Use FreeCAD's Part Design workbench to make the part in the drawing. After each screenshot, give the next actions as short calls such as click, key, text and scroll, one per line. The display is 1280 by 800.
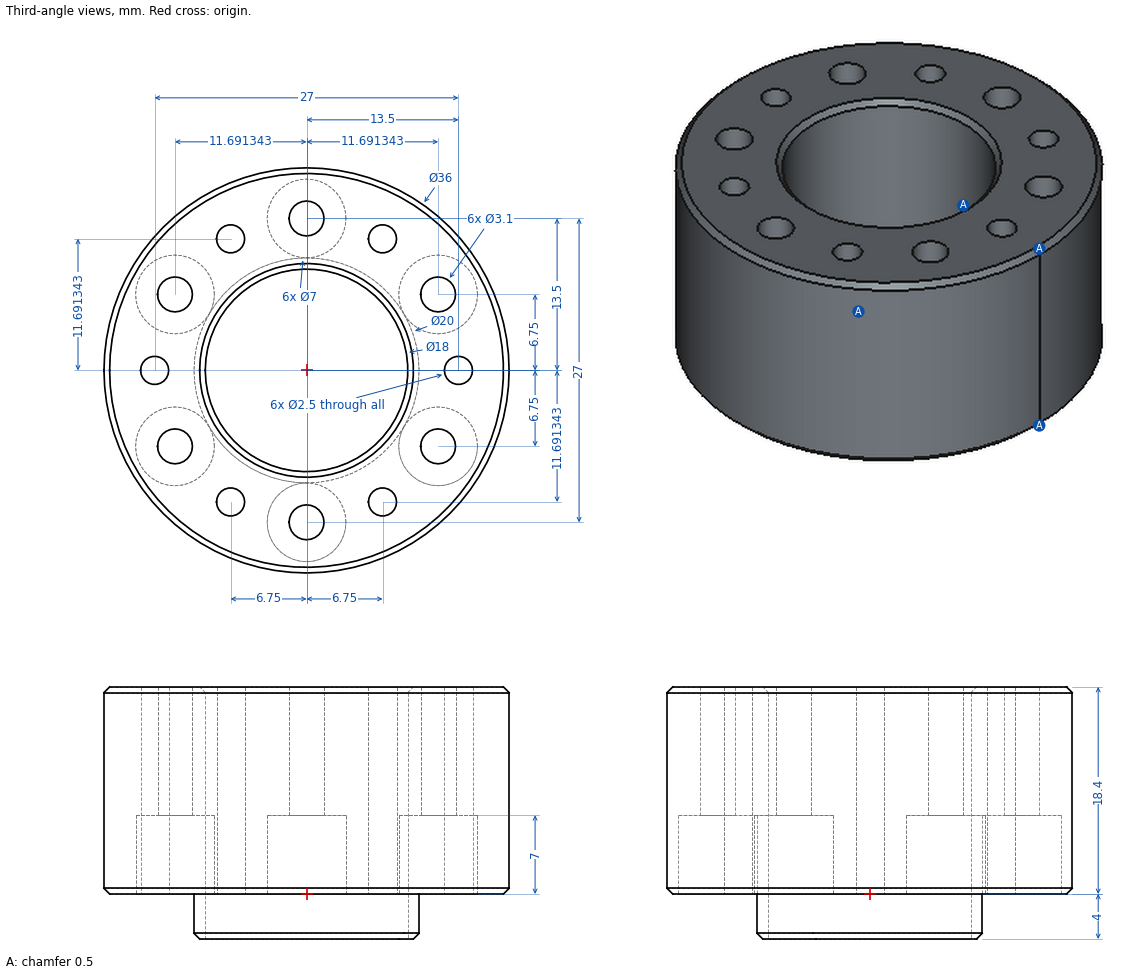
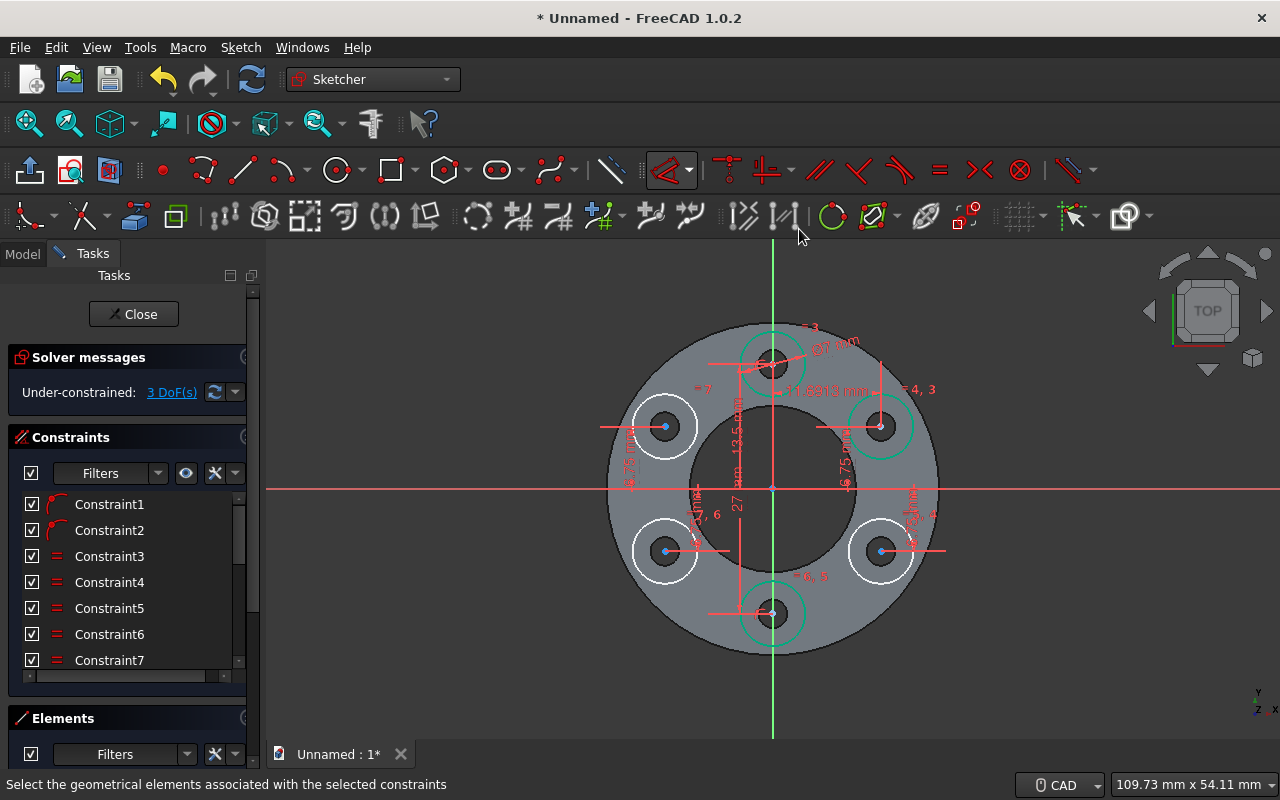
click(881, 551)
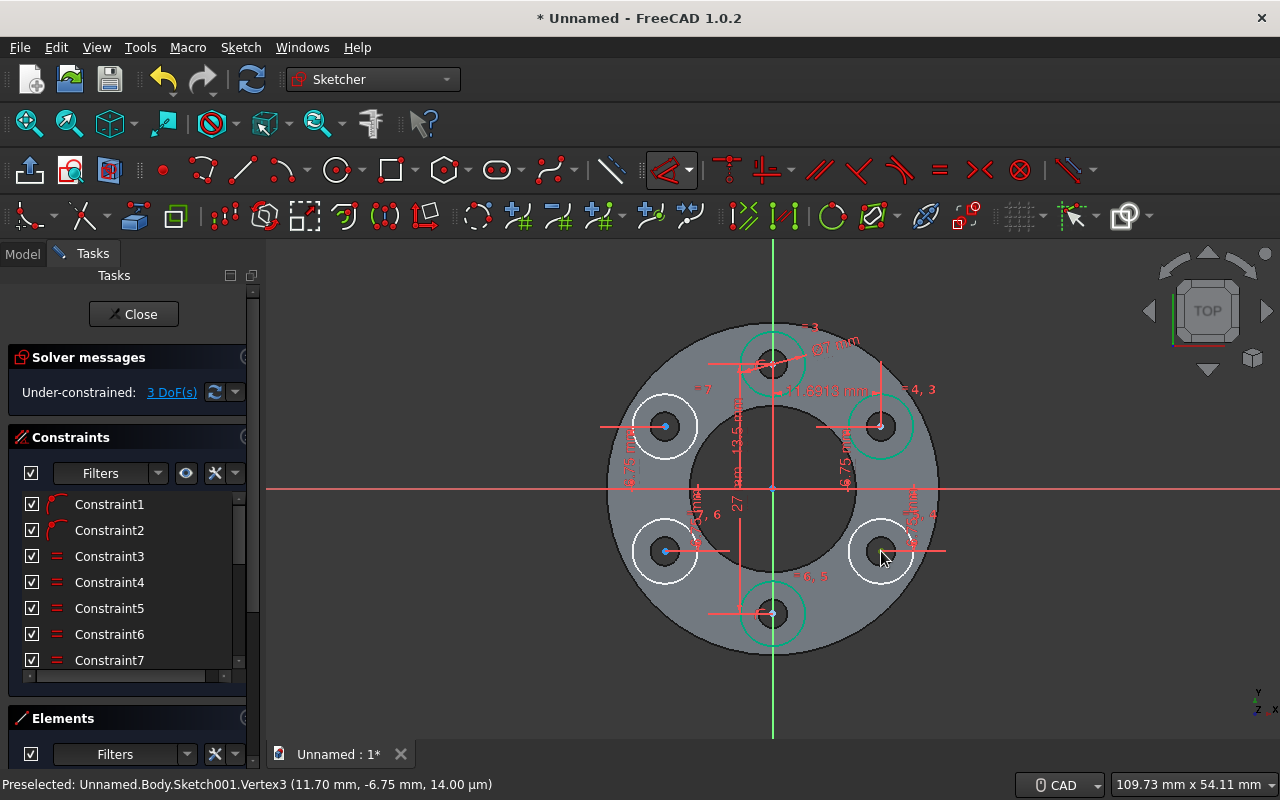
key(l)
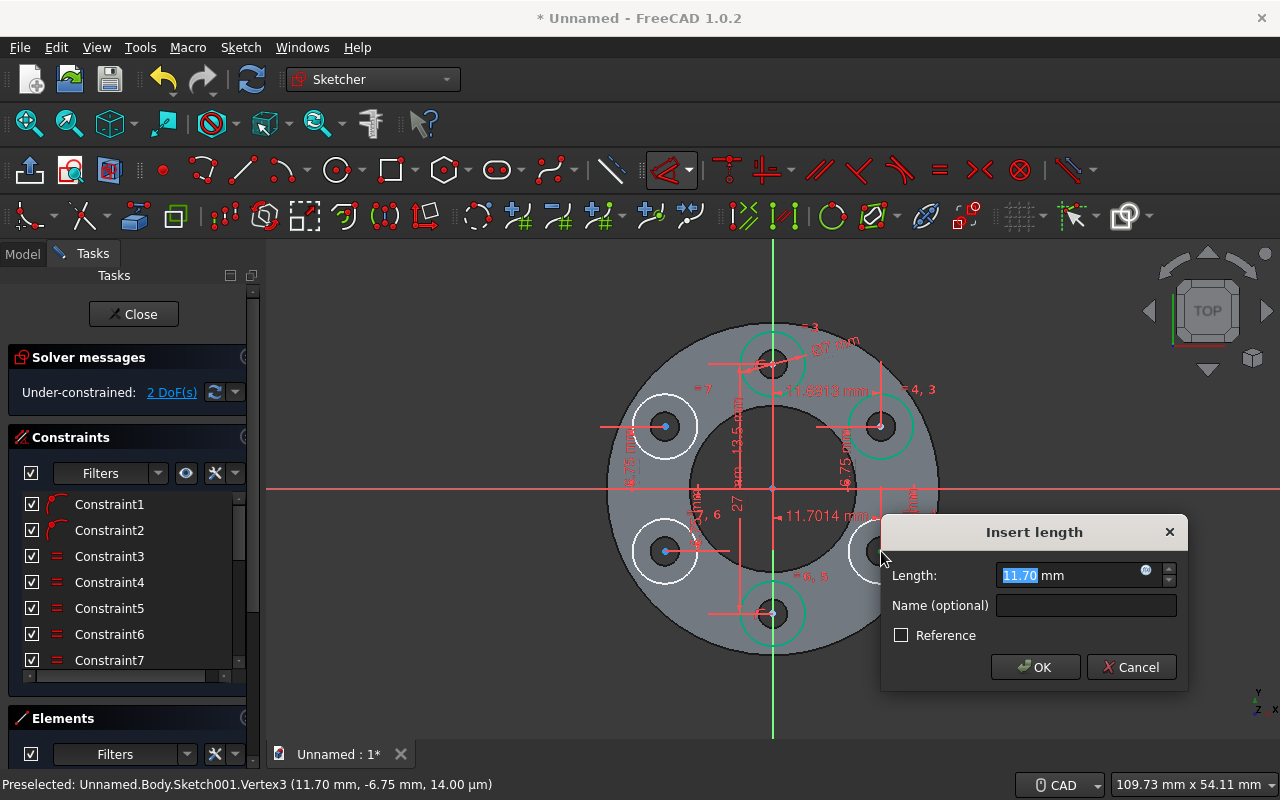
text(11.691343)
key(Return)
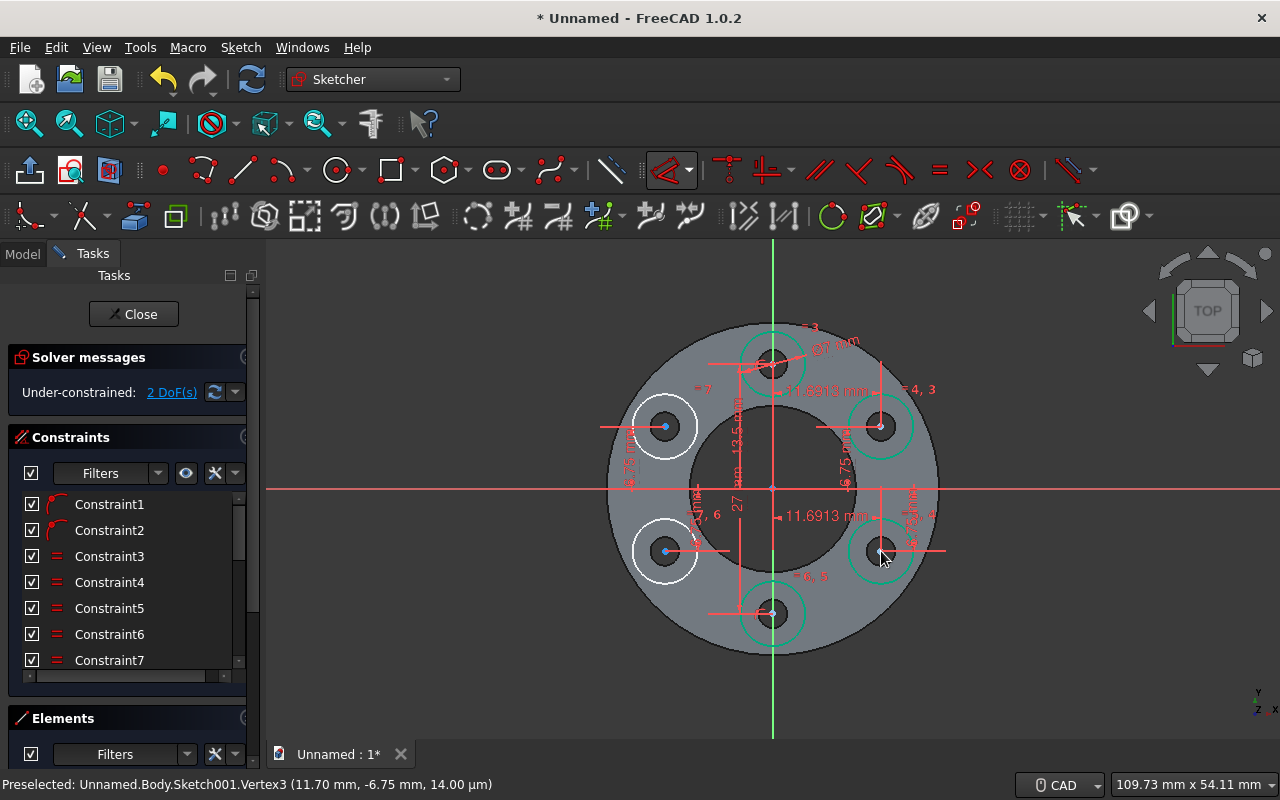
click(665, 551)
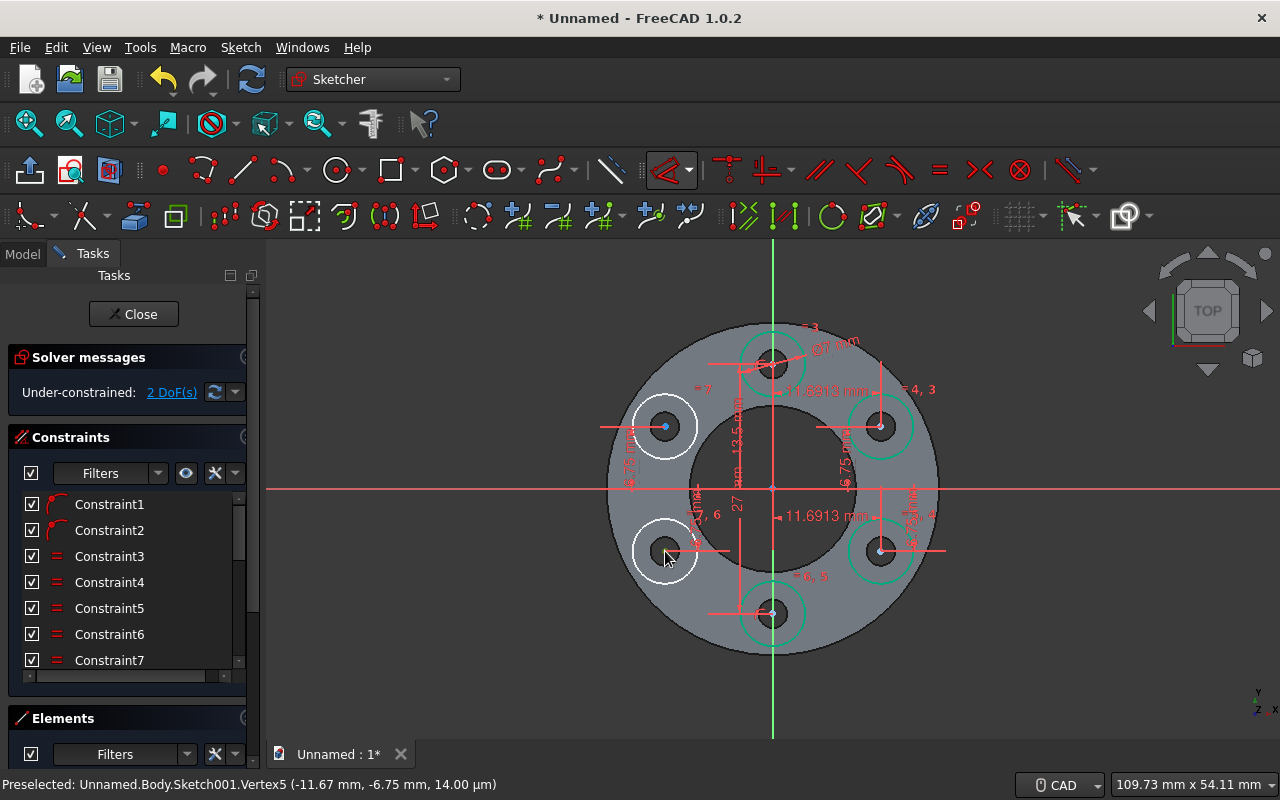
click(692, 170)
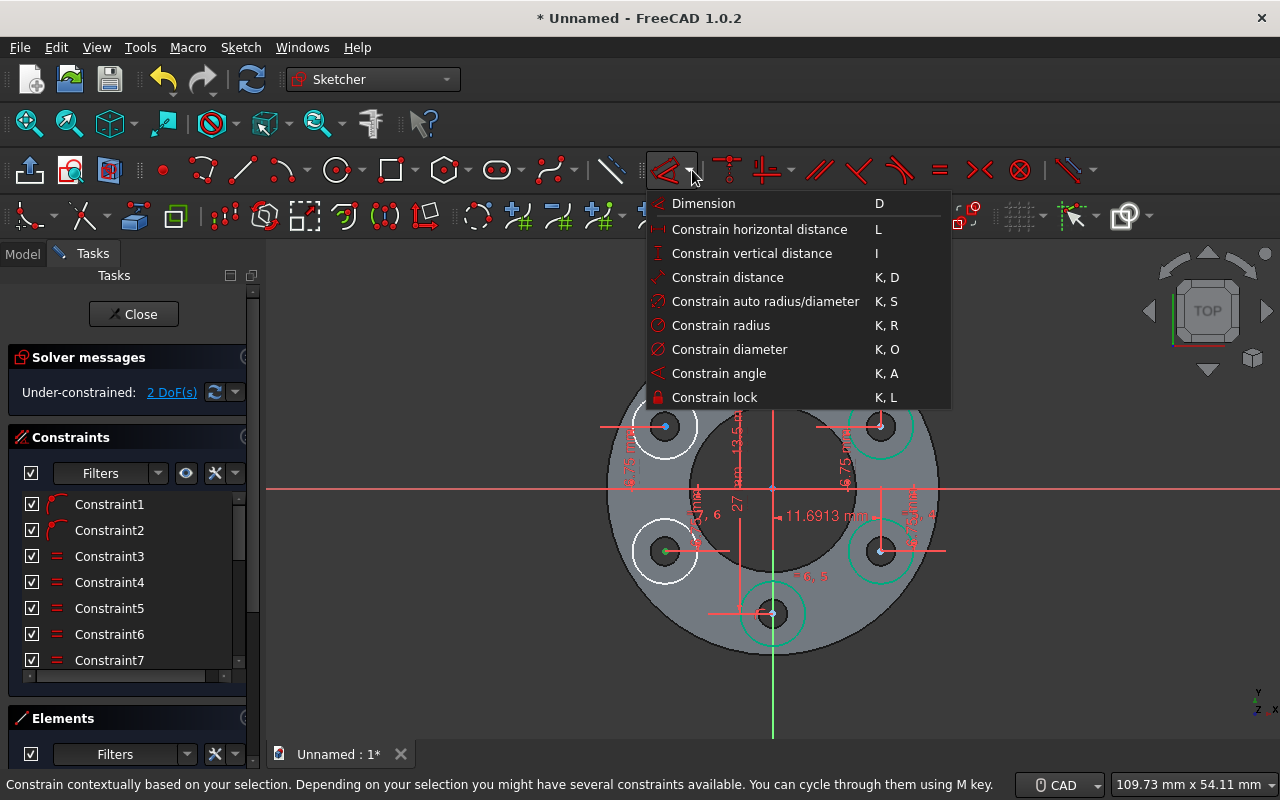
click(799, 229)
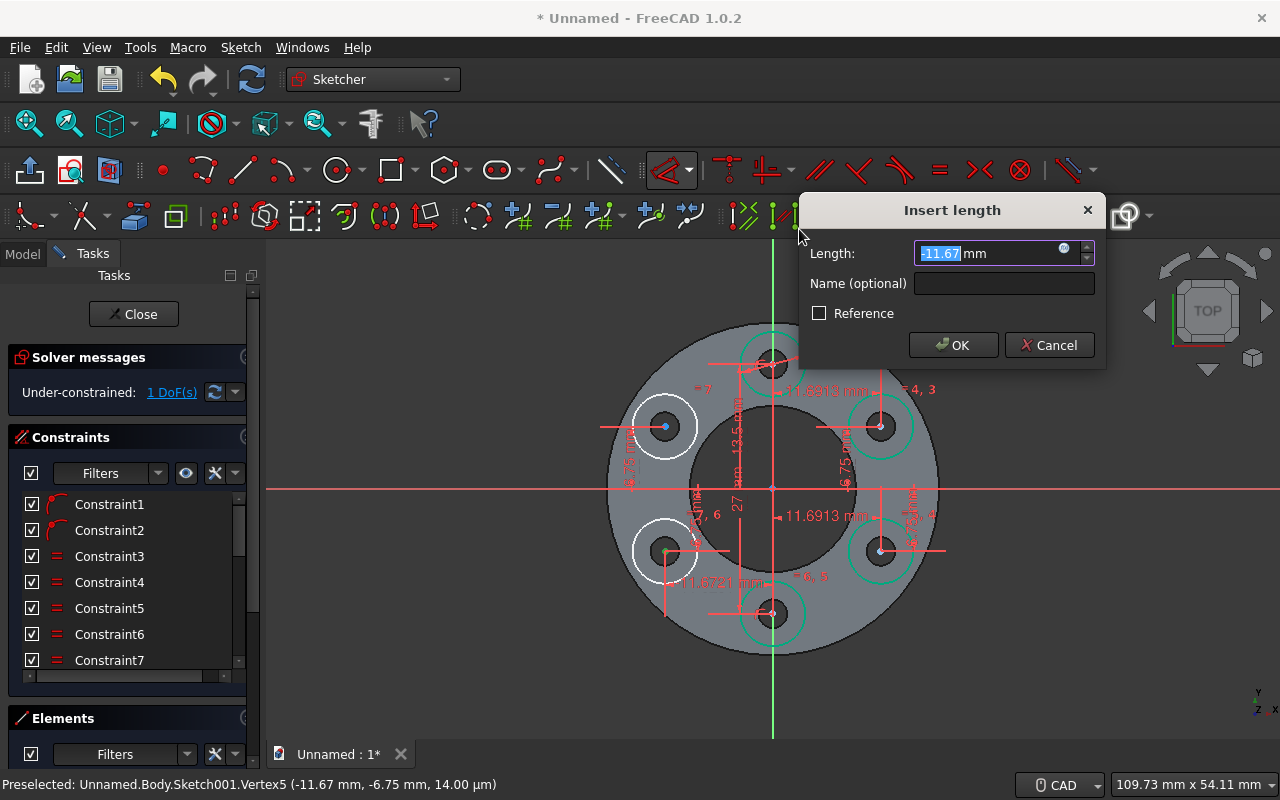
text(-11.691343)
key(Return)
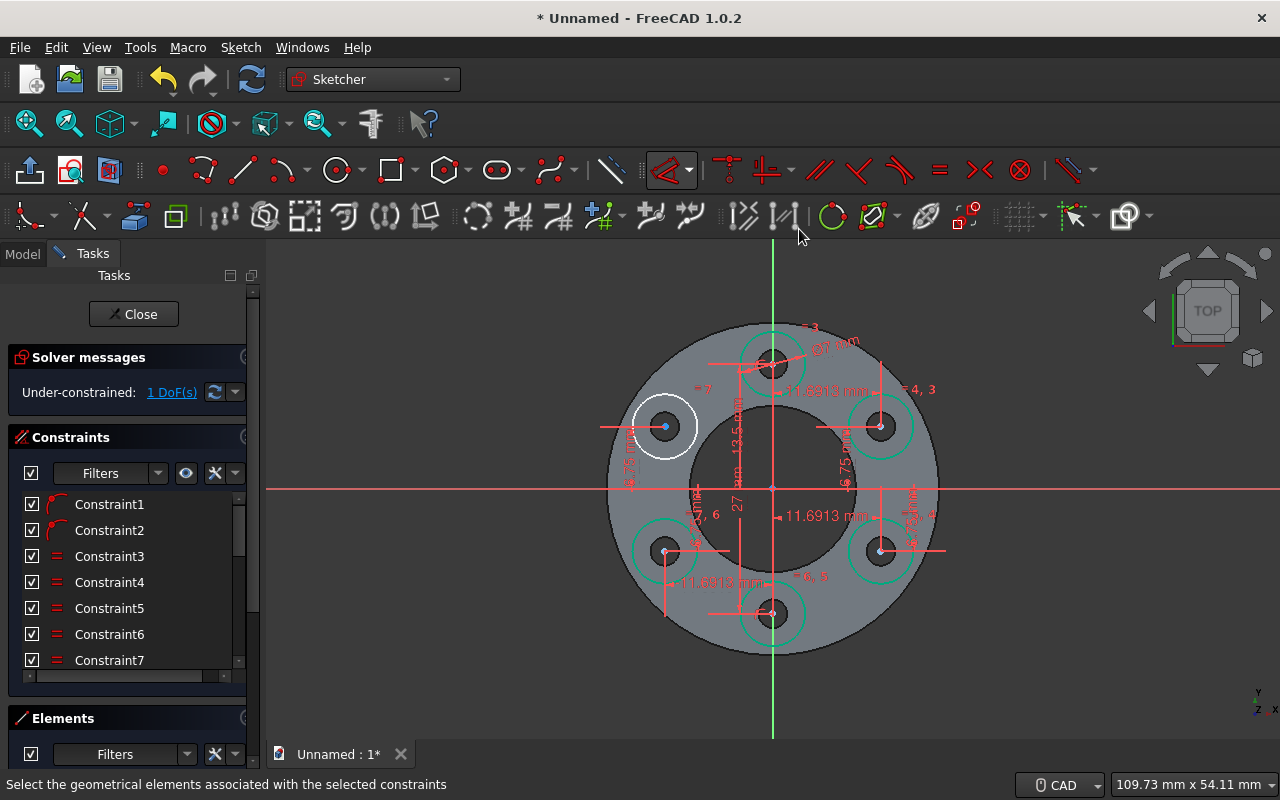
click(665, 427)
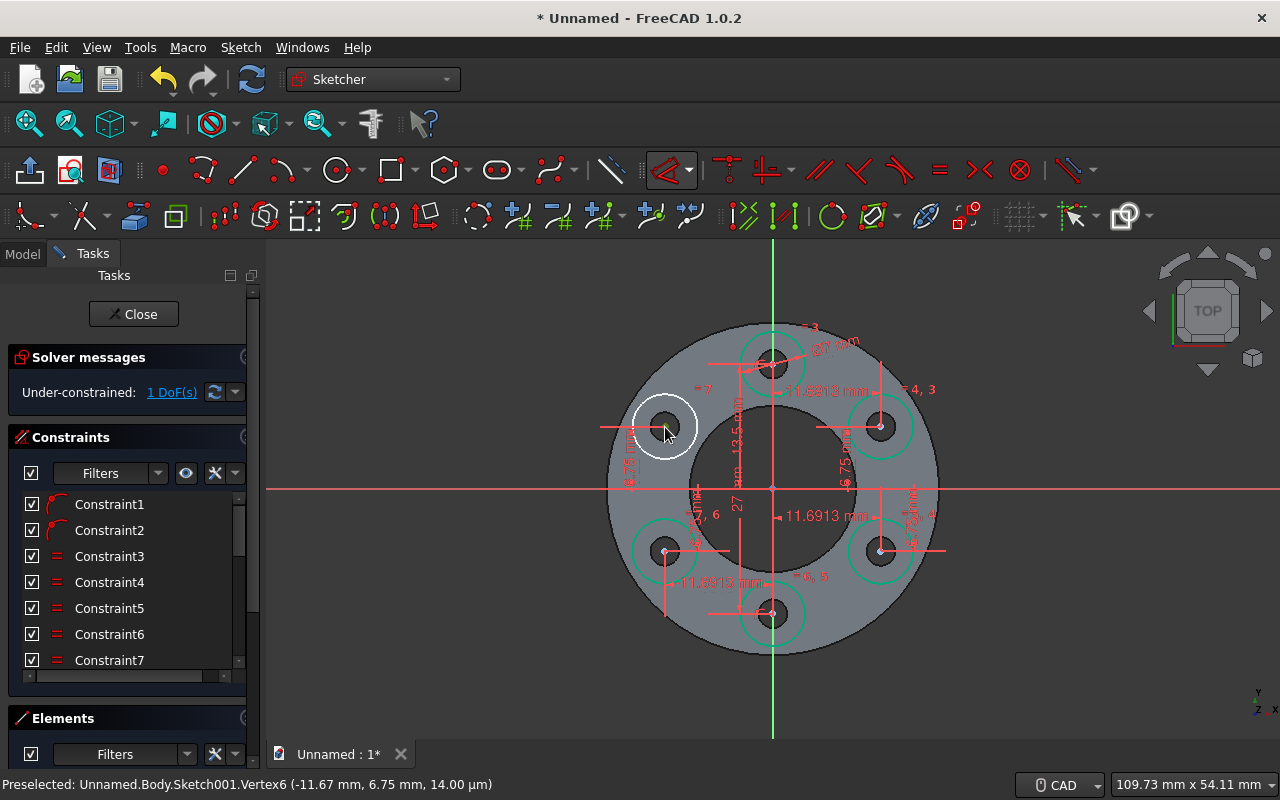
click(692, 170)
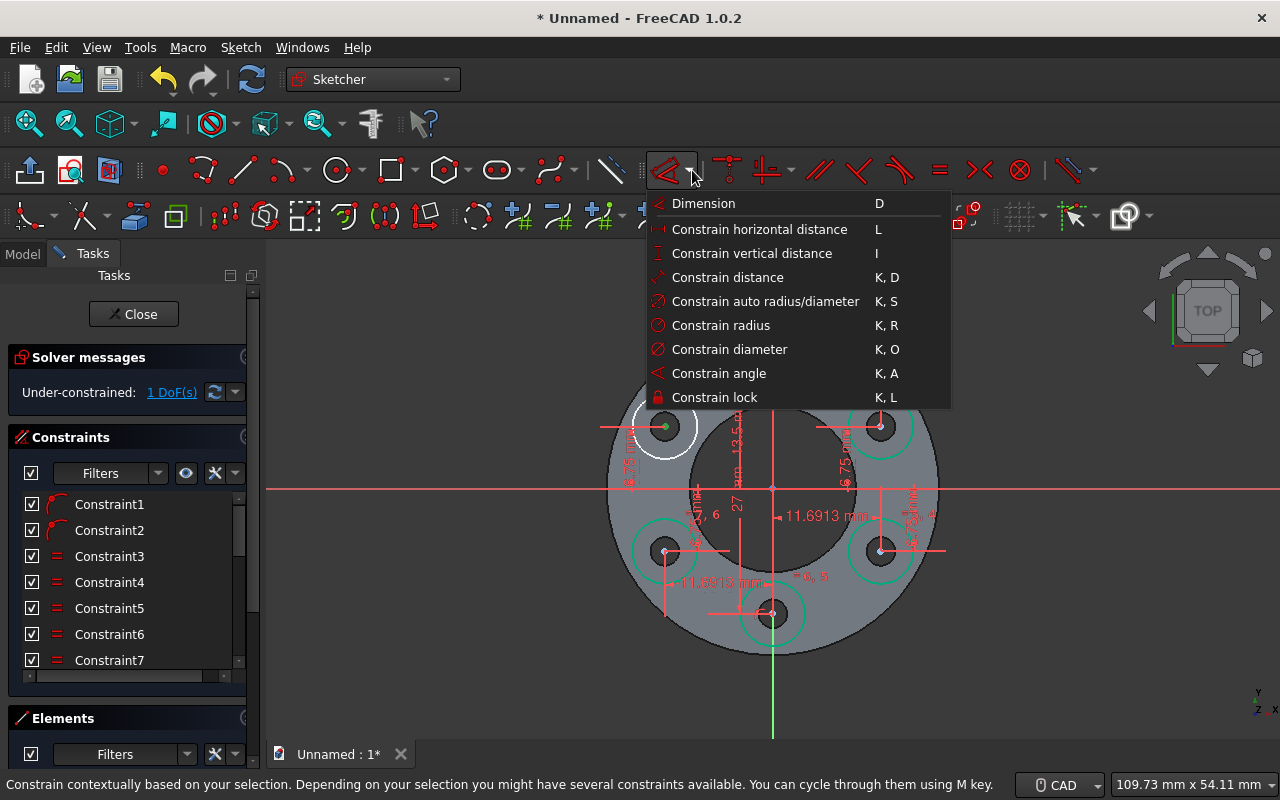
click(799, 229)